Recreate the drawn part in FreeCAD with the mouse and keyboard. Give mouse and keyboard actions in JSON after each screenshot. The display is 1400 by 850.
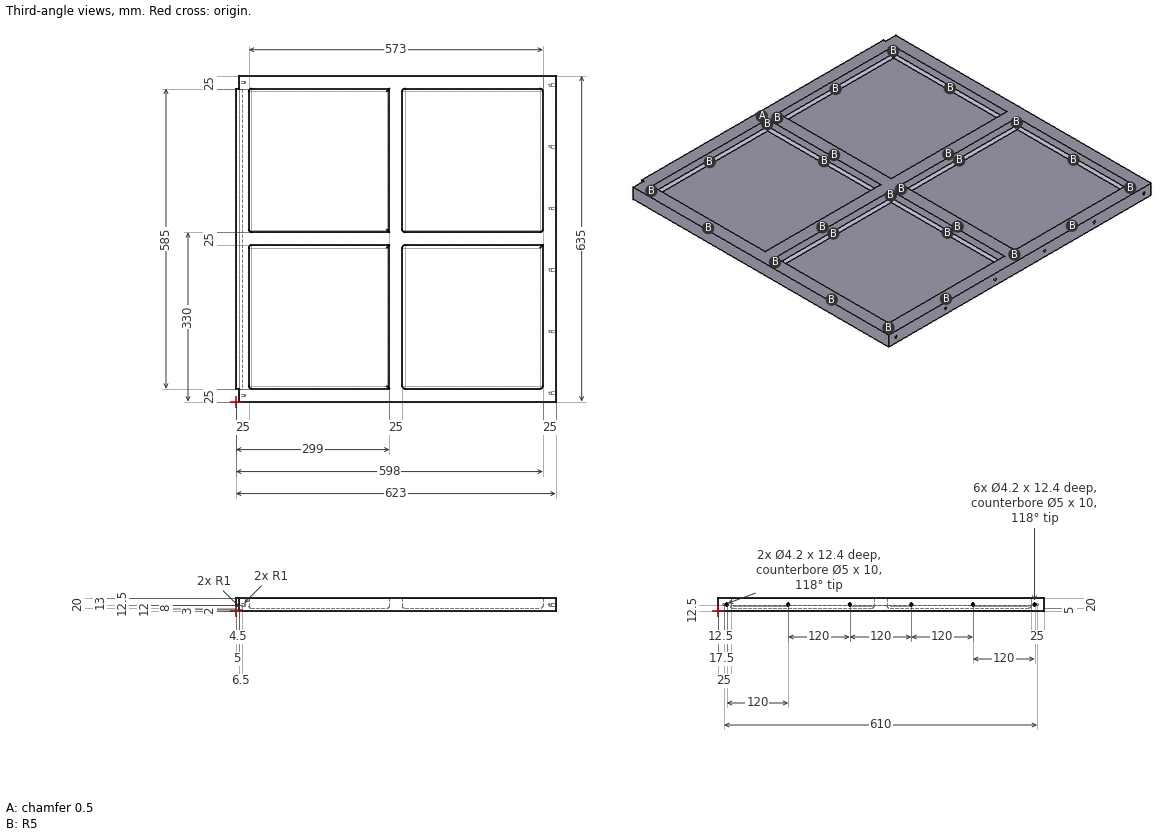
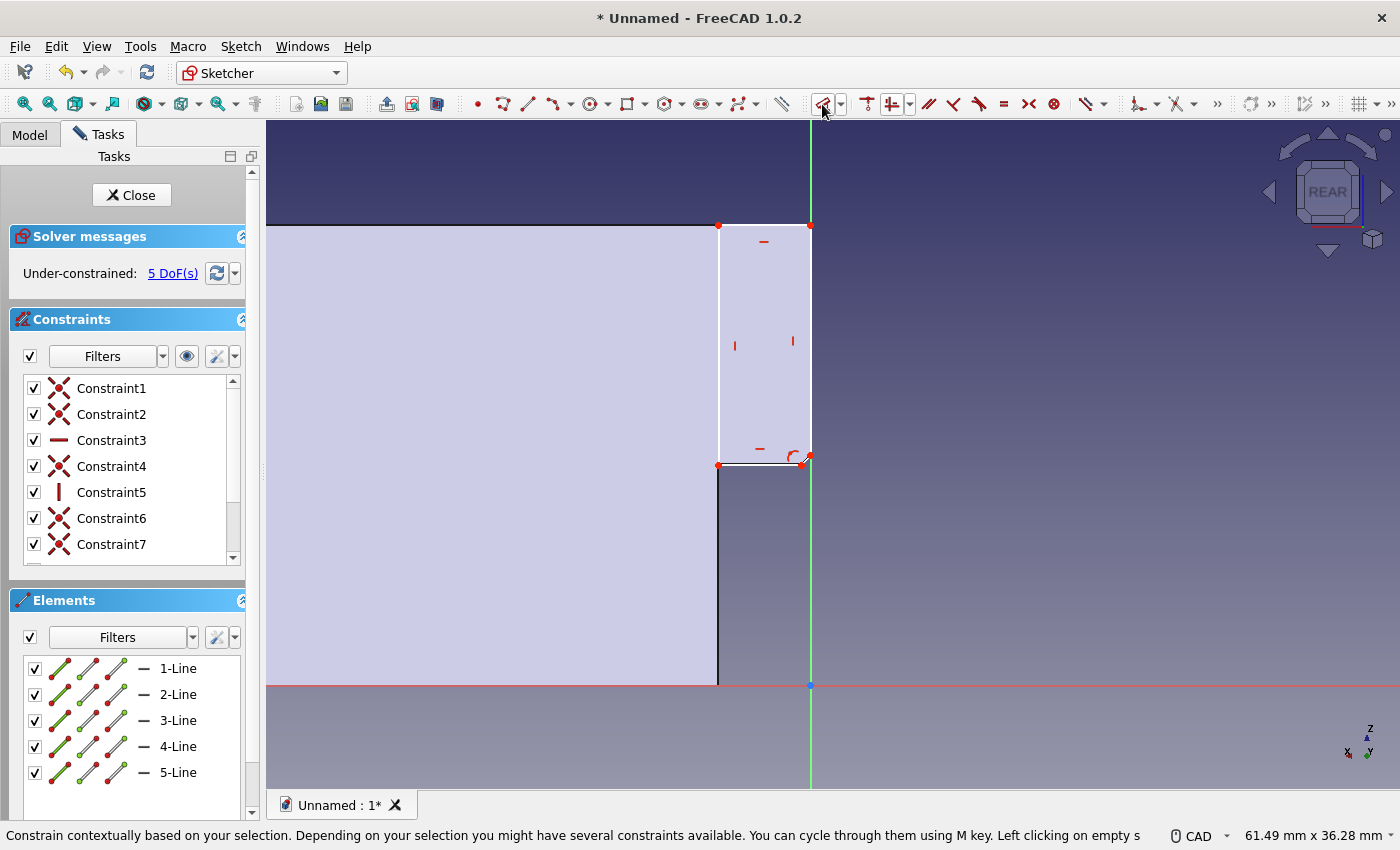
{"action": "left_click", "coordinate": [783, 225]}
{"action": "left_click", "coordinate": [765, 191]}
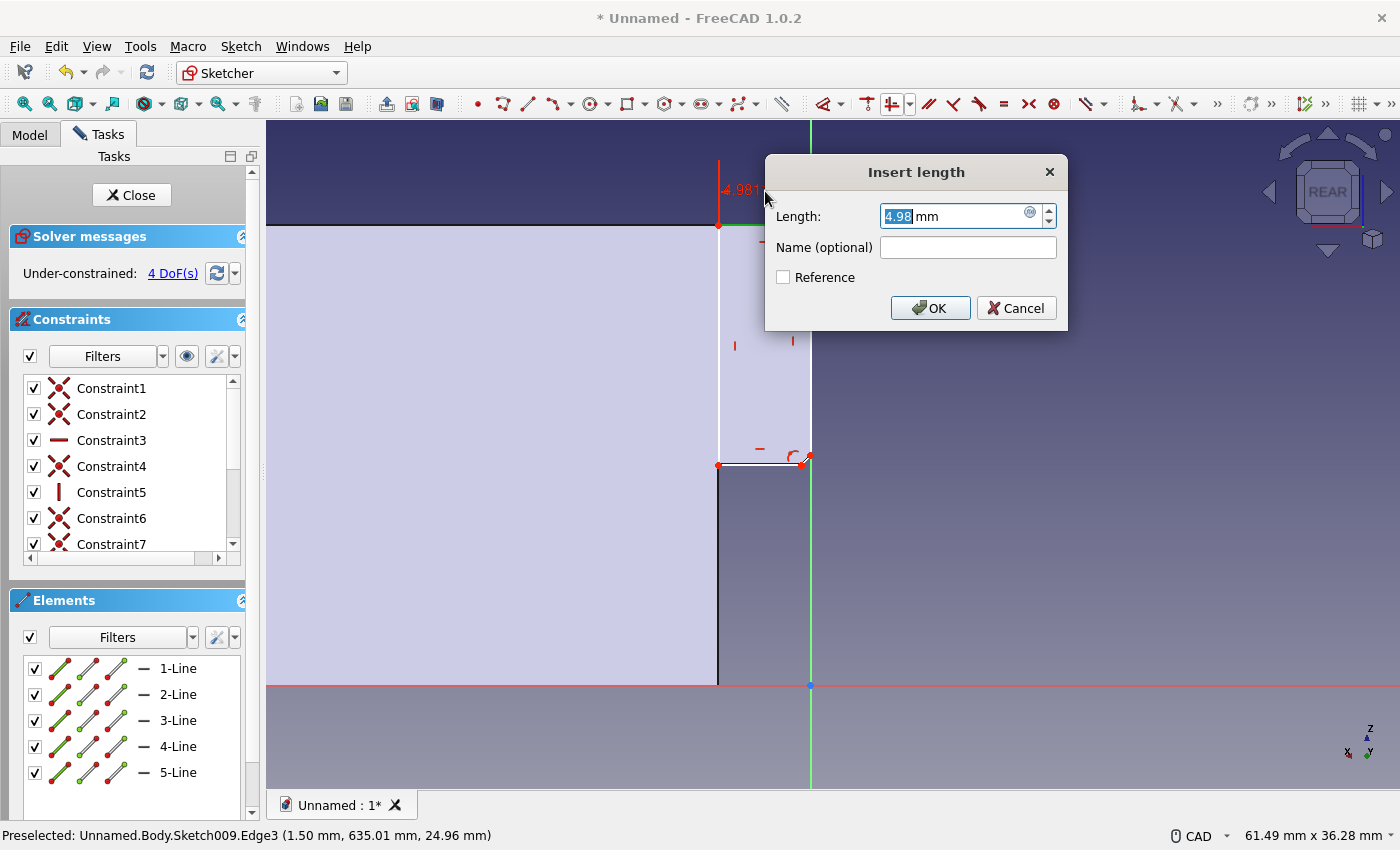
{"action": "type", "text": "5"}
{"action": "key", "text": "Return"}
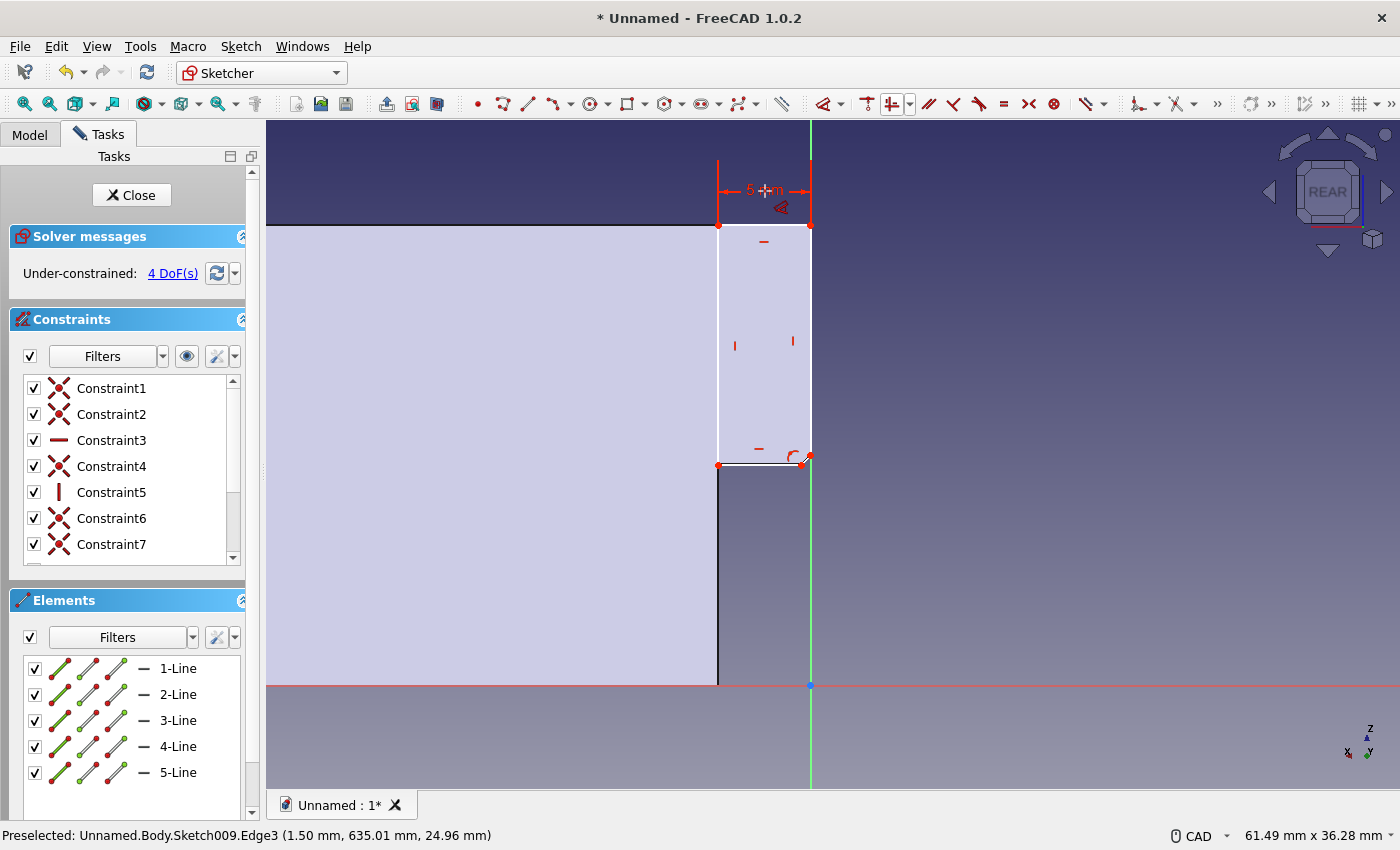
{"action": "left_click", "coordinate": [718, 297]}
{"action": "left_click", "coordinate": [684, 345]}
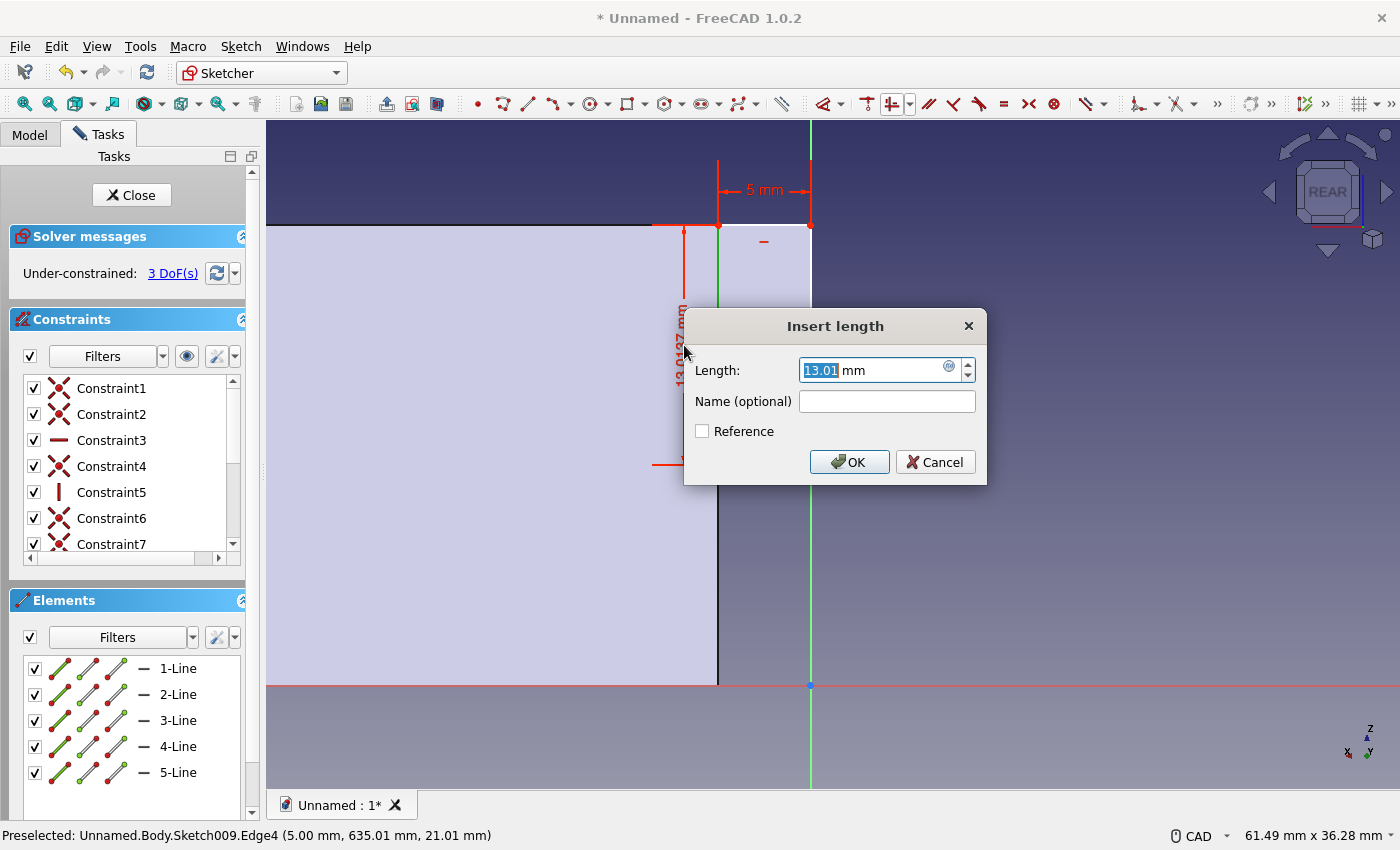
{"action": "type", "text": "13"}
{"action": "key", "text": "Return"}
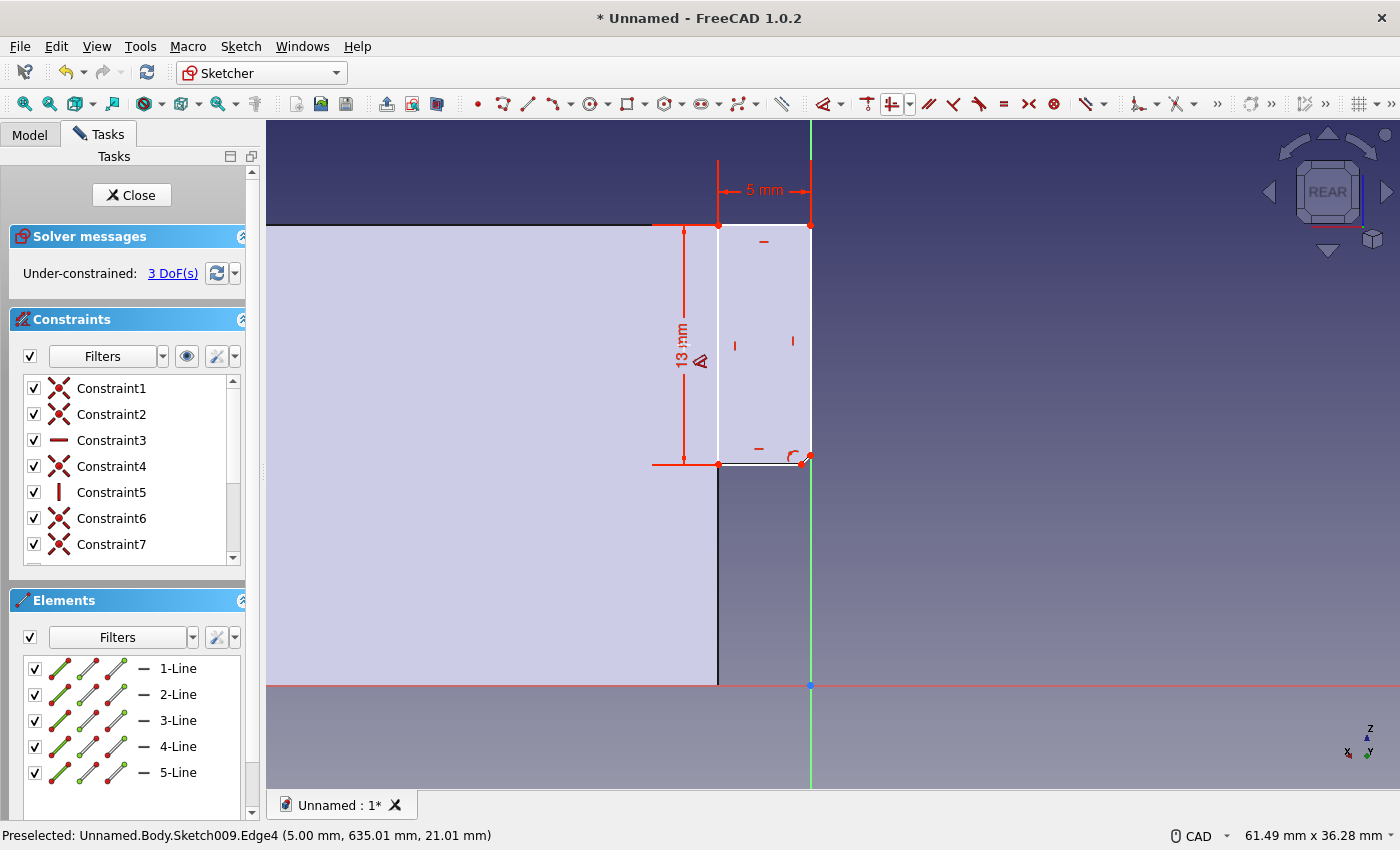
{"action": "left_click", "coordinate": [743, 465]}
{"action": "left_click", "coordinate": [760, 499]}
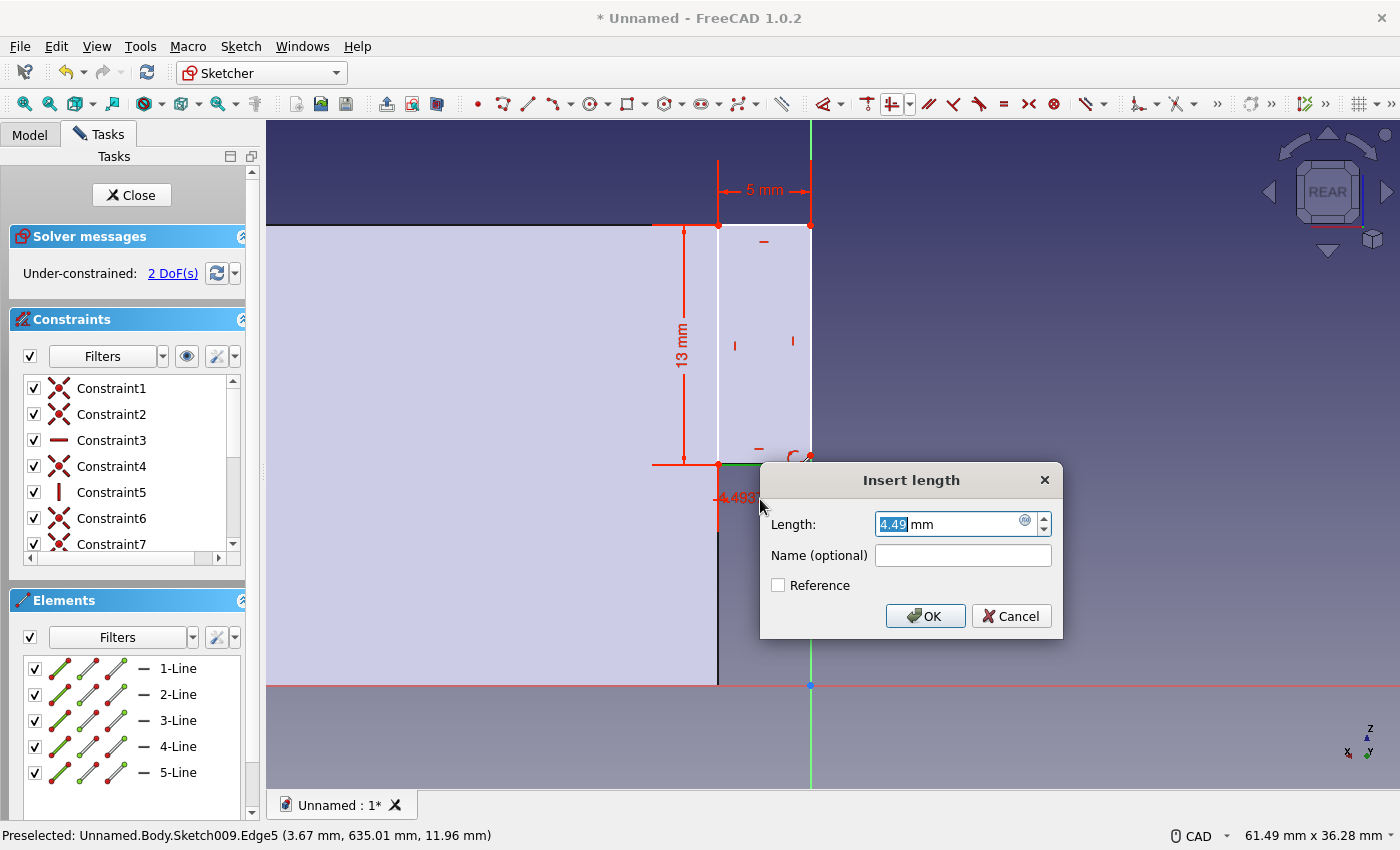
{"action": "type", "text": "4.5"}
{"action": "key", "text": "Return"}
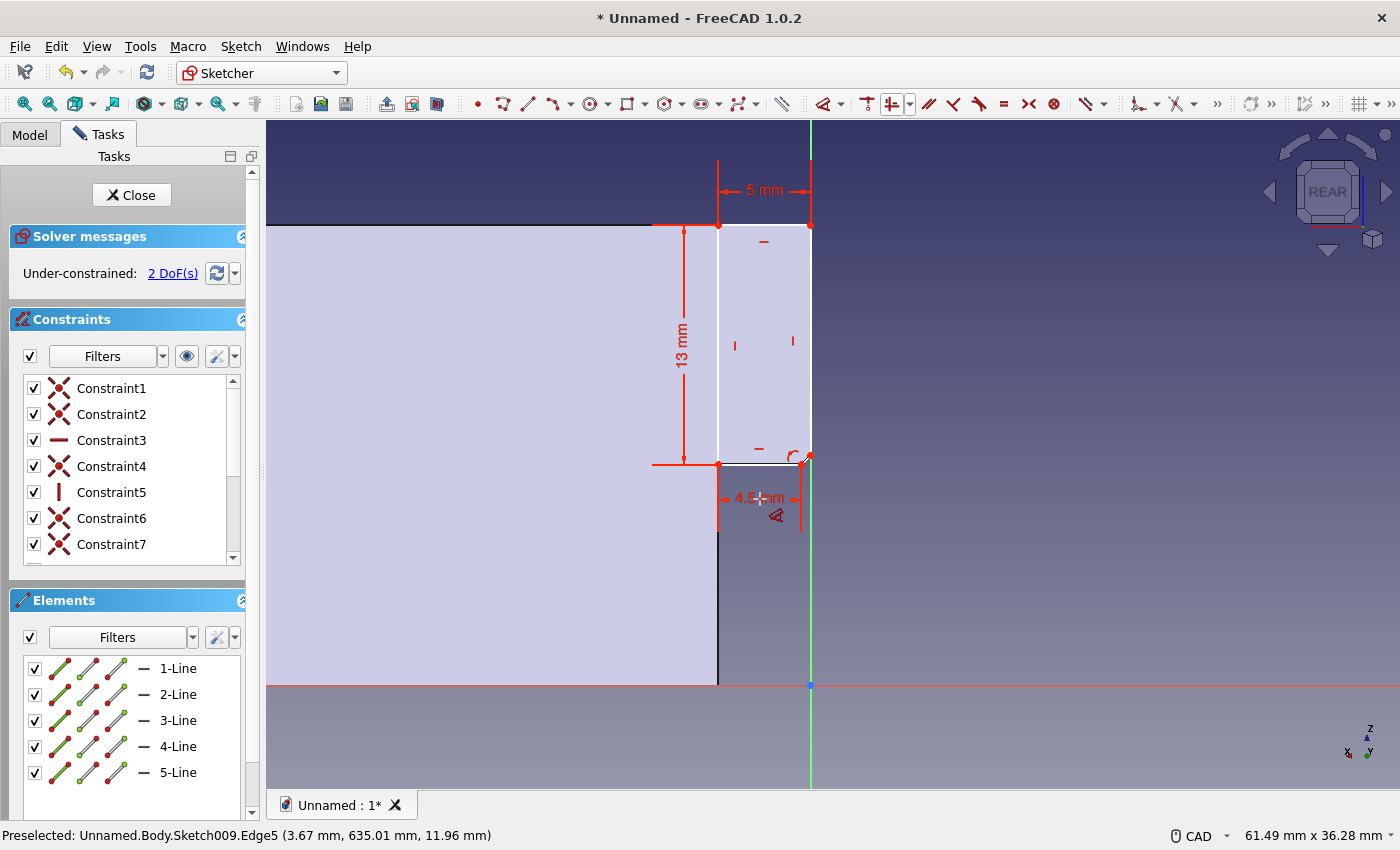
{"action": "left_click", "coordinate": [801, 465]}
{"action": "left_click", "coordinate": [845, 575]}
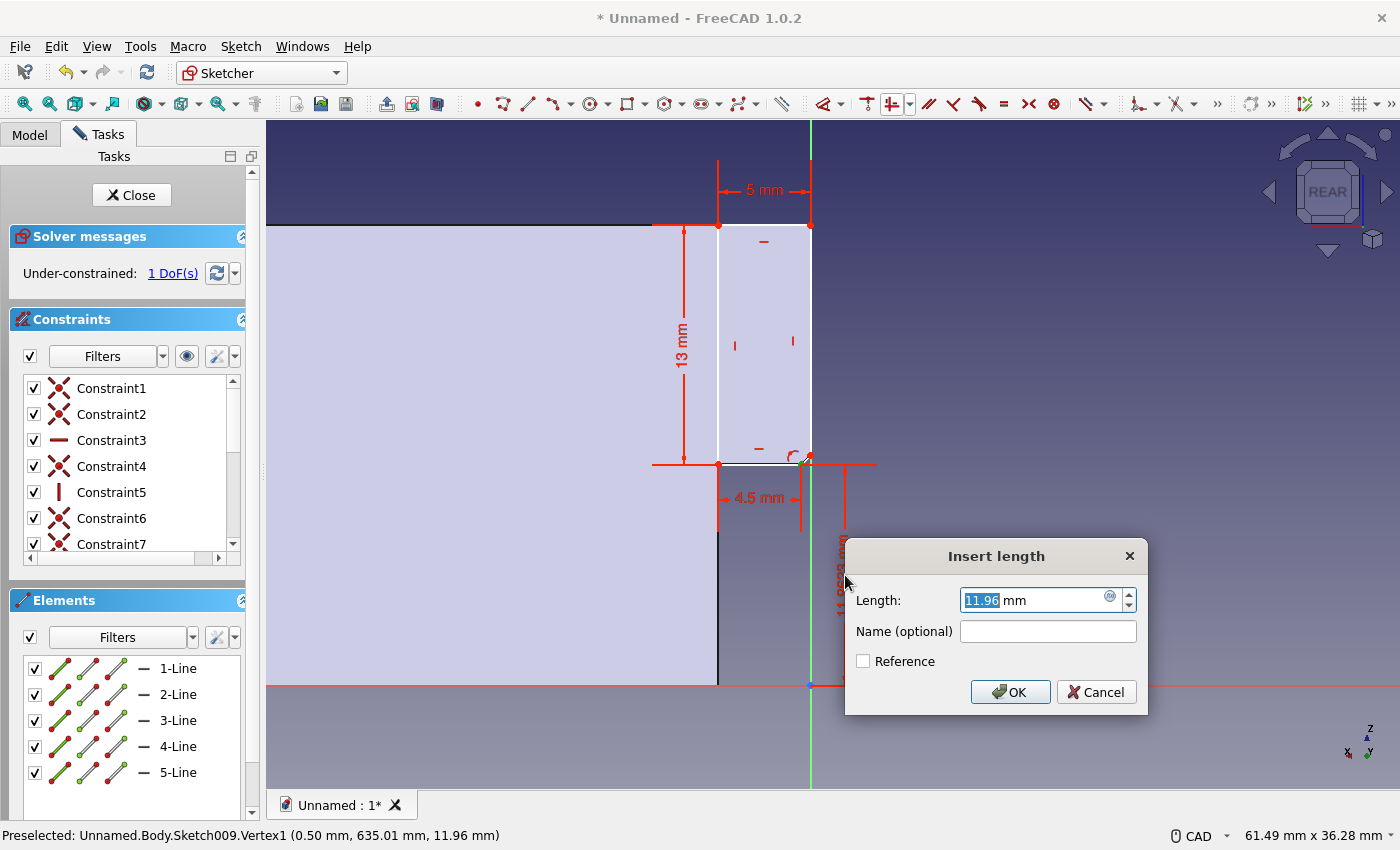
{"action": "type", "text": "12"}
{"action": "key", "text": "Return"}